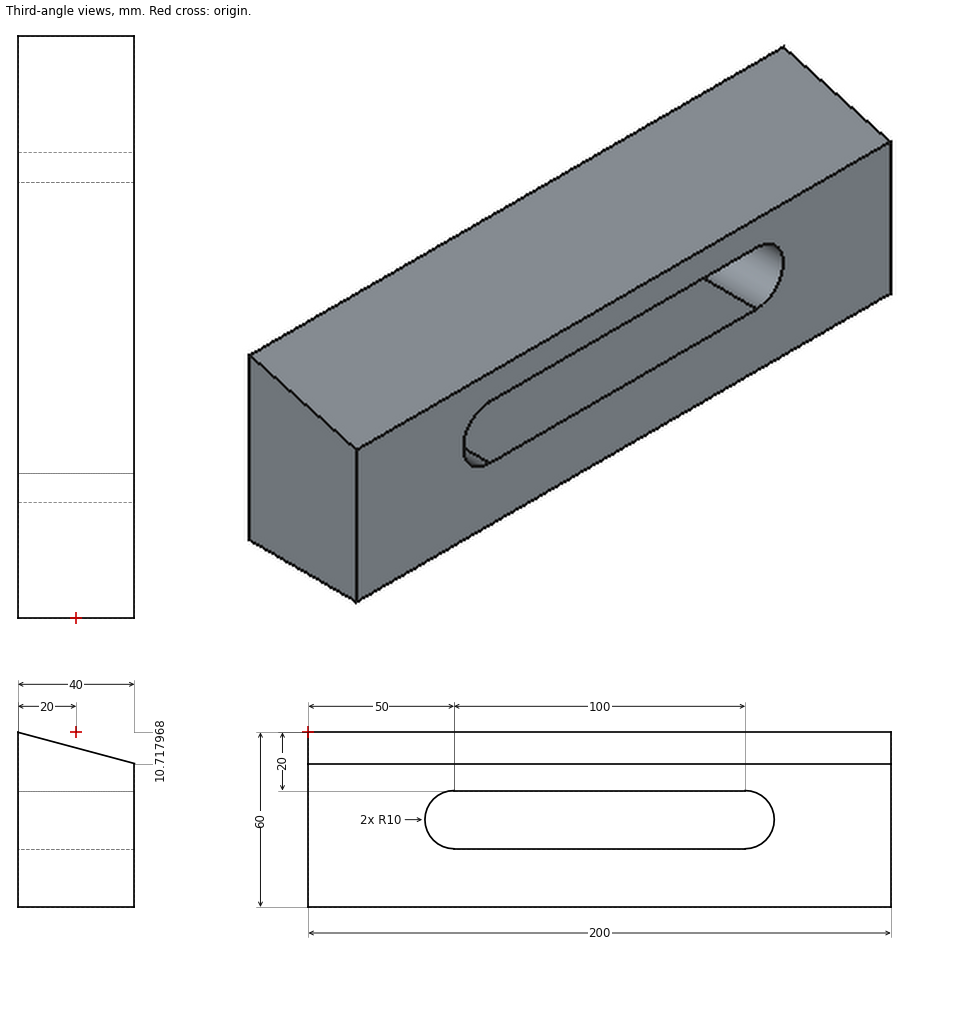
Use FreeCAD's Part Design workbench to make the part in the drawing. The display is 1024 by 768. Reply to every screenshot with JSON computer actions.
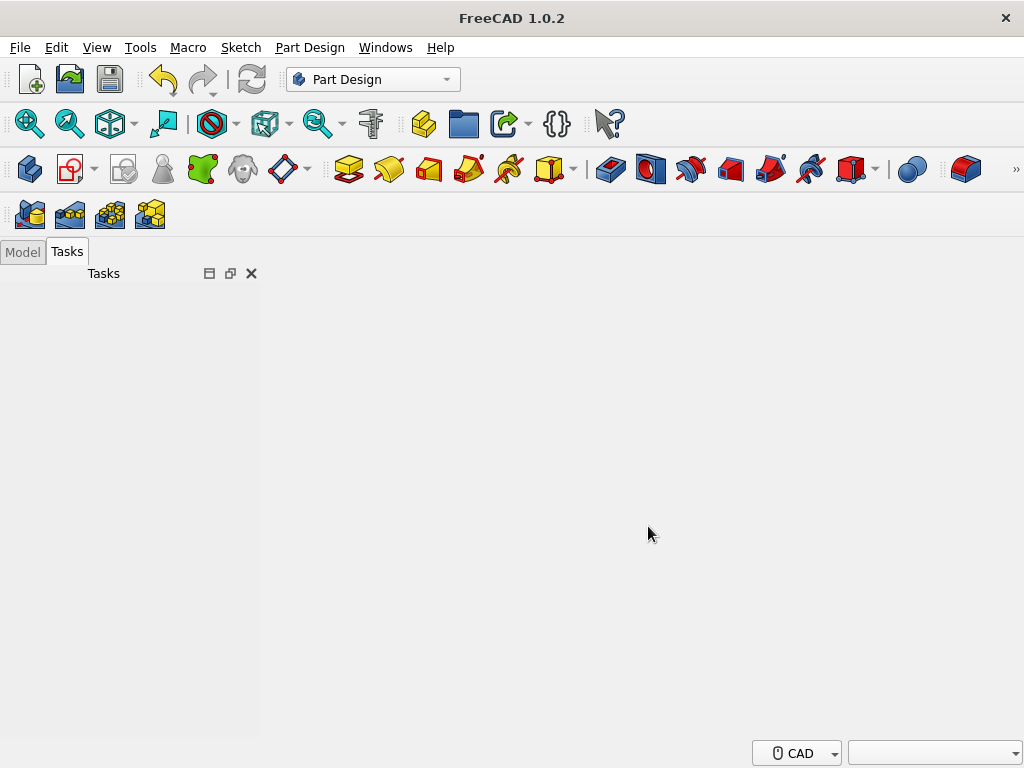
{"action": "left_click", "coordinate": [30, 80]}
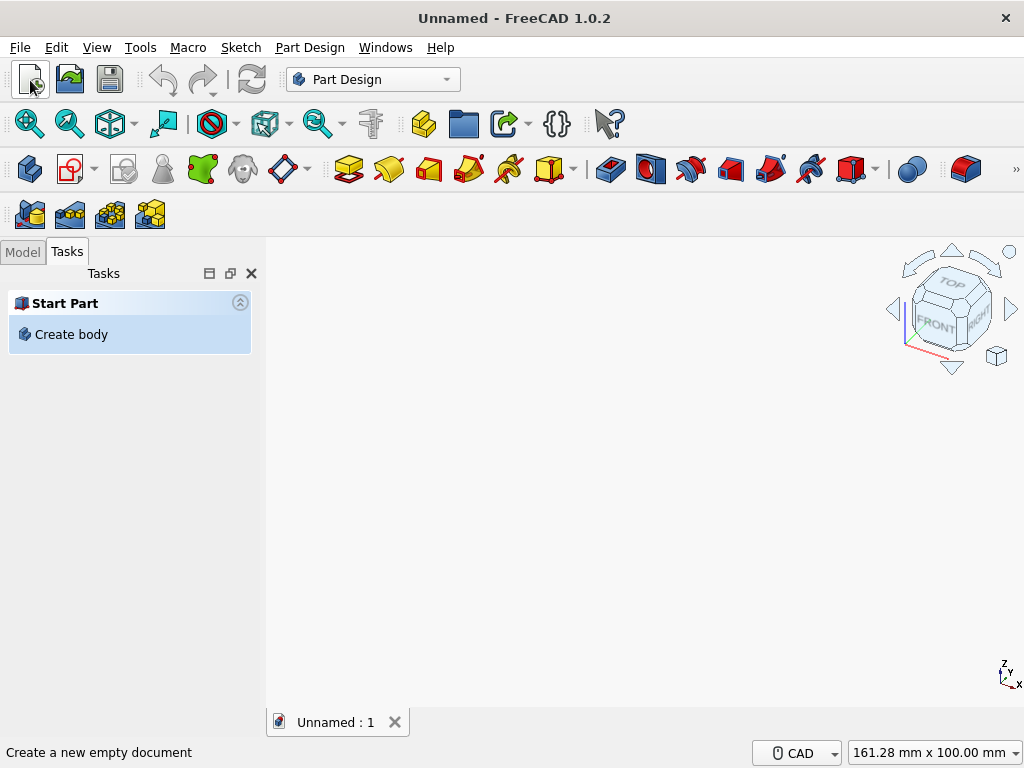
{"action": "left_click", "coordinate": [70, 170]}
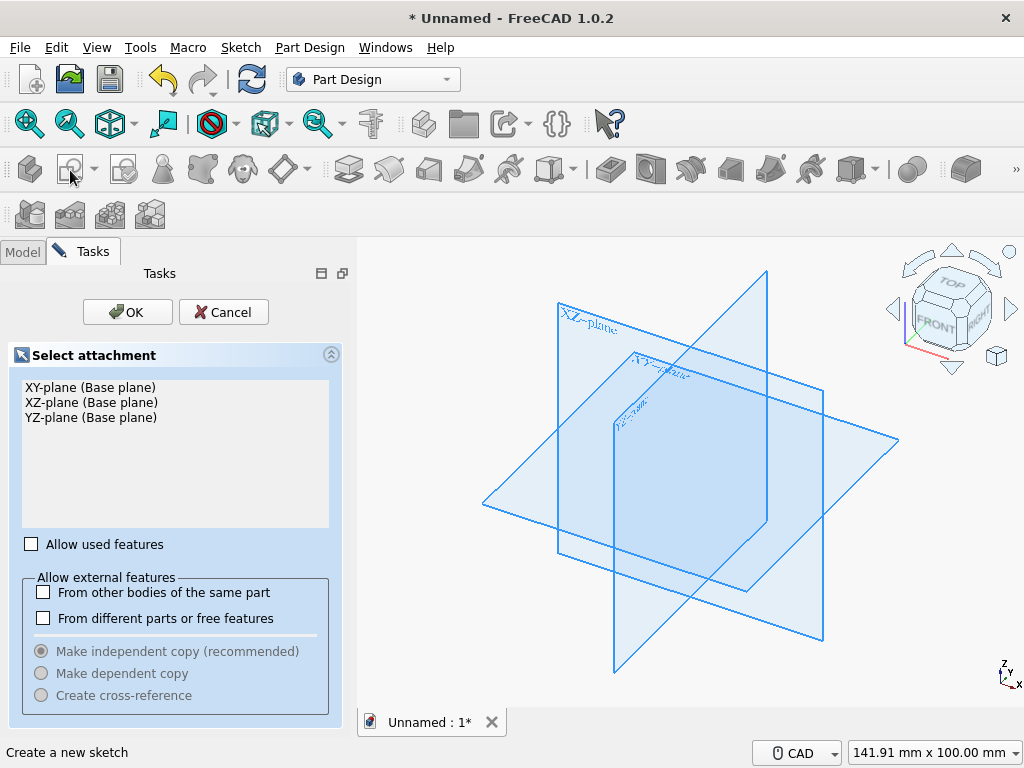
{"action": "left_click", "coordinate": [82, 418]}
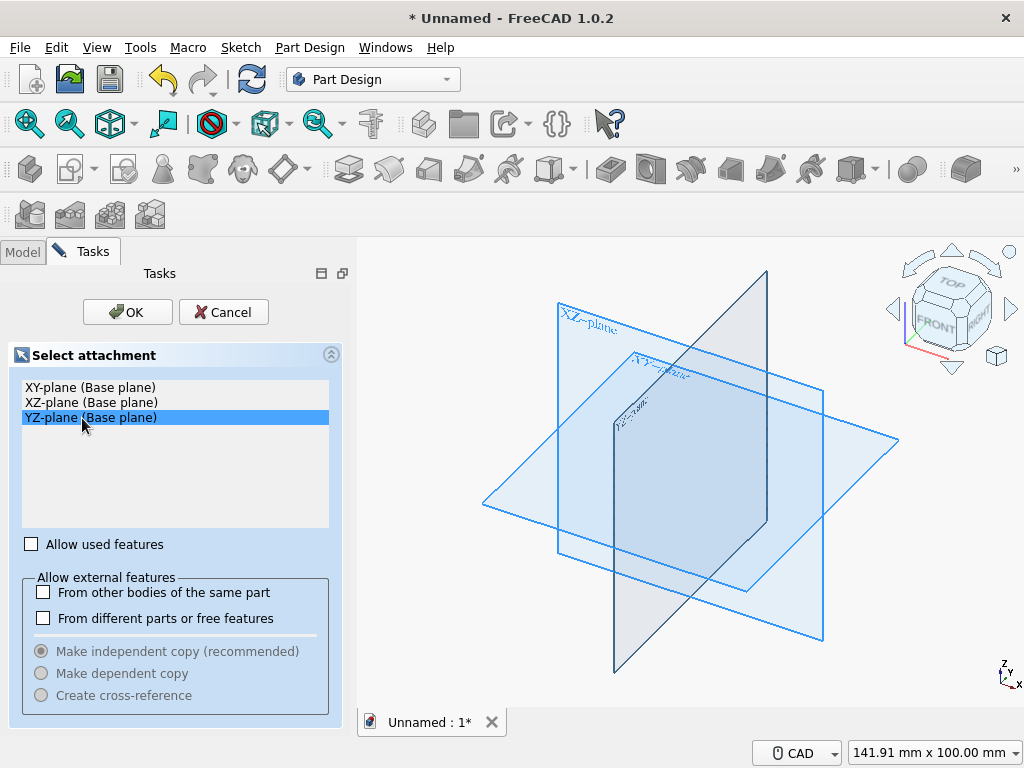
{"action": "left_click", "coordinate": [128, 312]}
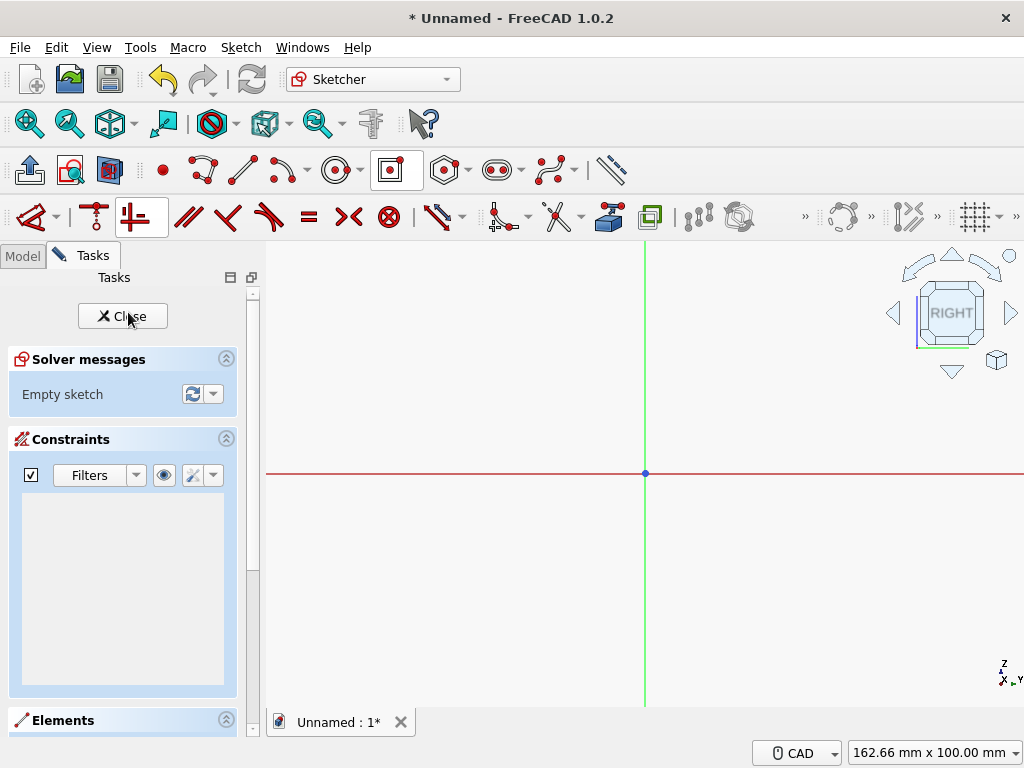
{"action": "scroll", "coordinate": [294, 393], "scroll_direction": "down", "scroll_amount": 5}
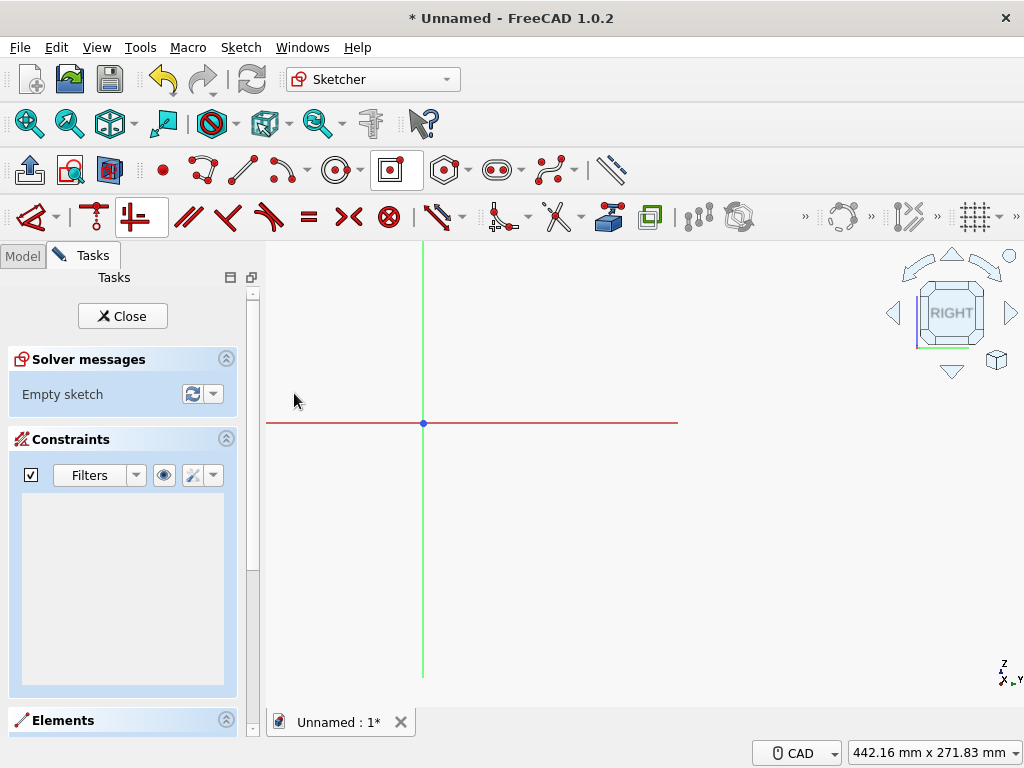
{"action": "left_click", "coordinate": [418, 170]}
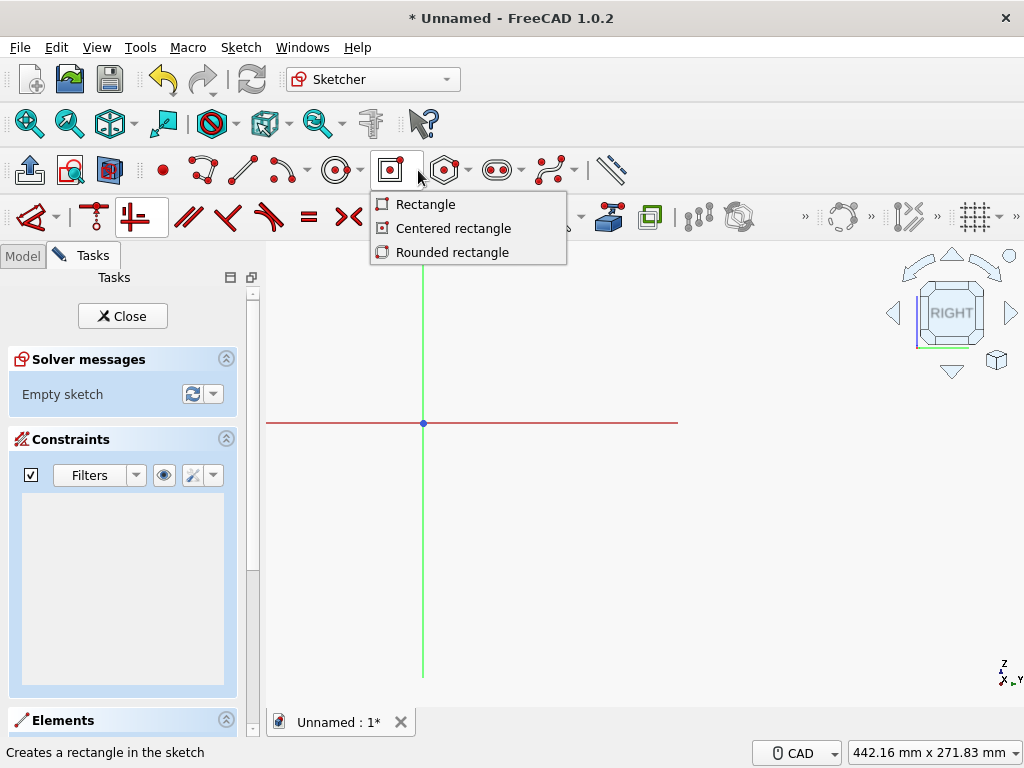
{"action": "left_click", "coordinate": [468, 204]}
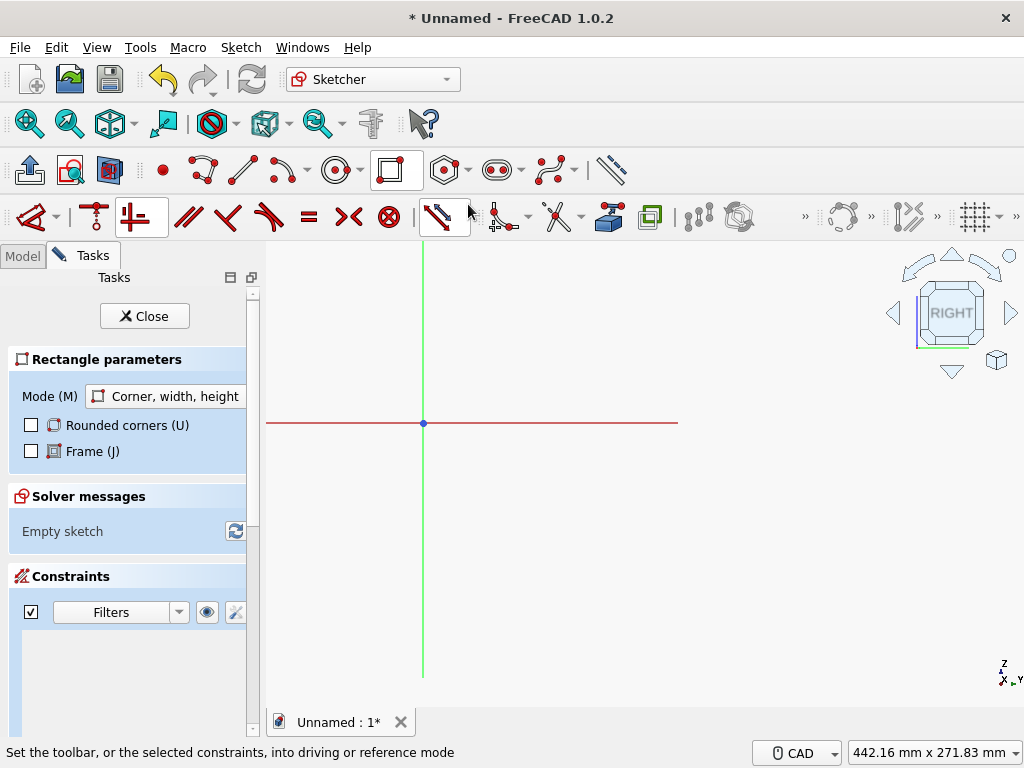
{"action": "left_click", "coordinate": [423, 423]}
{"action": "left_click", "coordinate": [766, 526]}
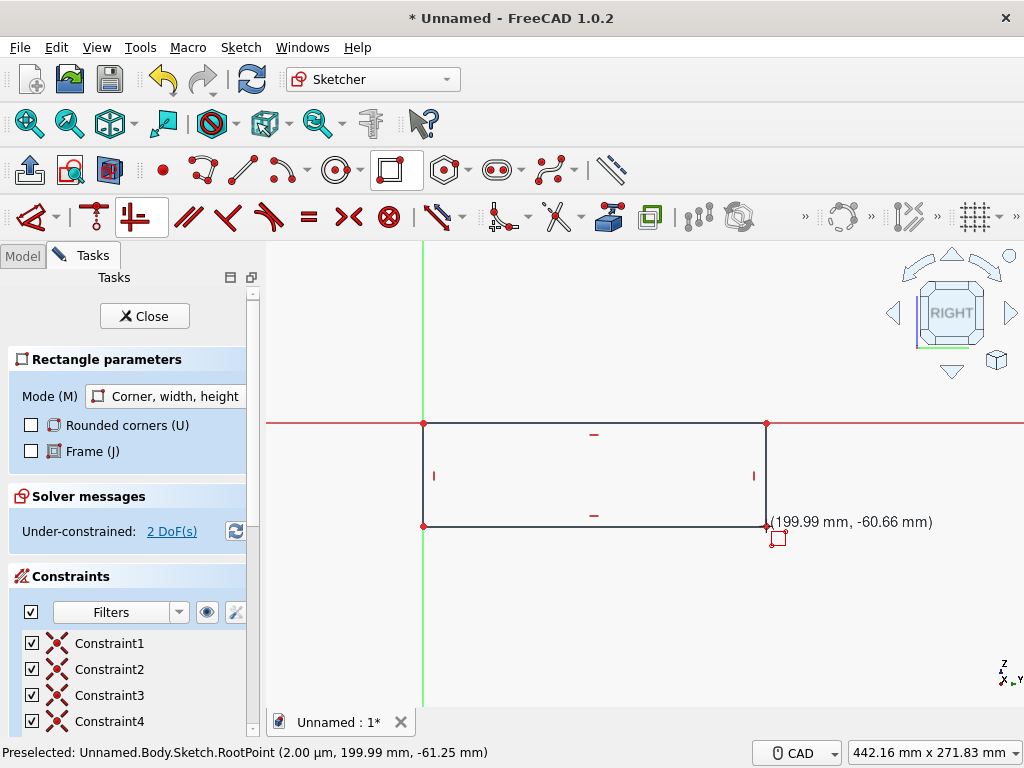
{"action": "left_click", "coordinate": [498, 170]}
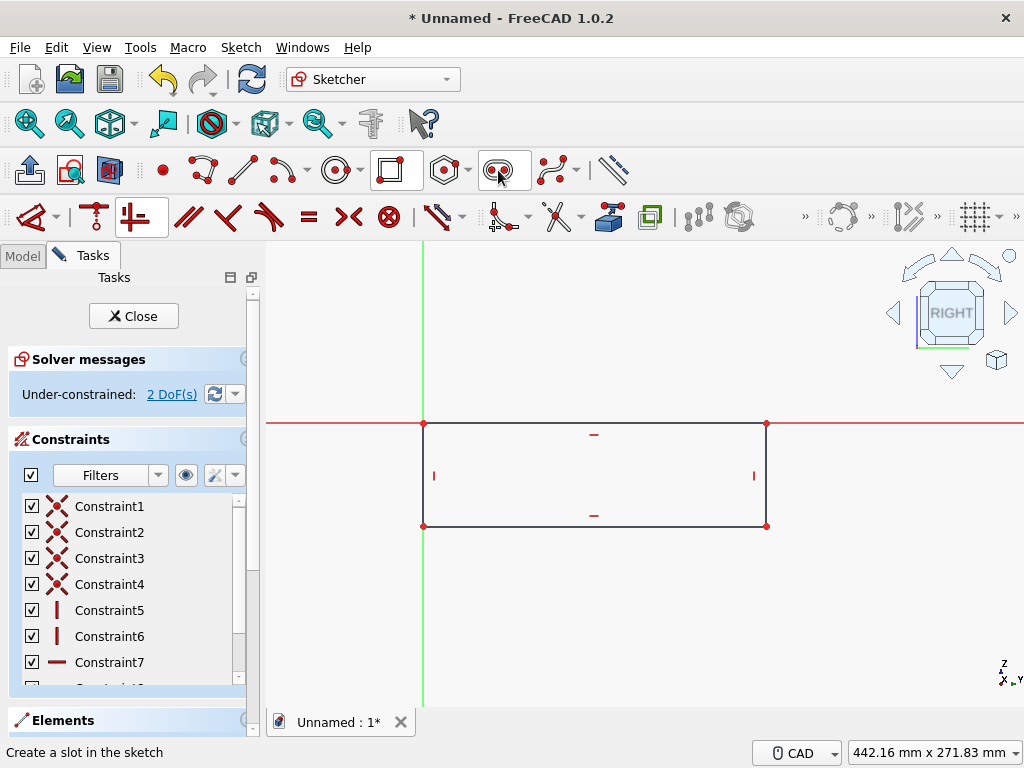
{"action": "scroll", "coordinate": [509, 474], "scroll_direction": "up", "scroll_amount": 2}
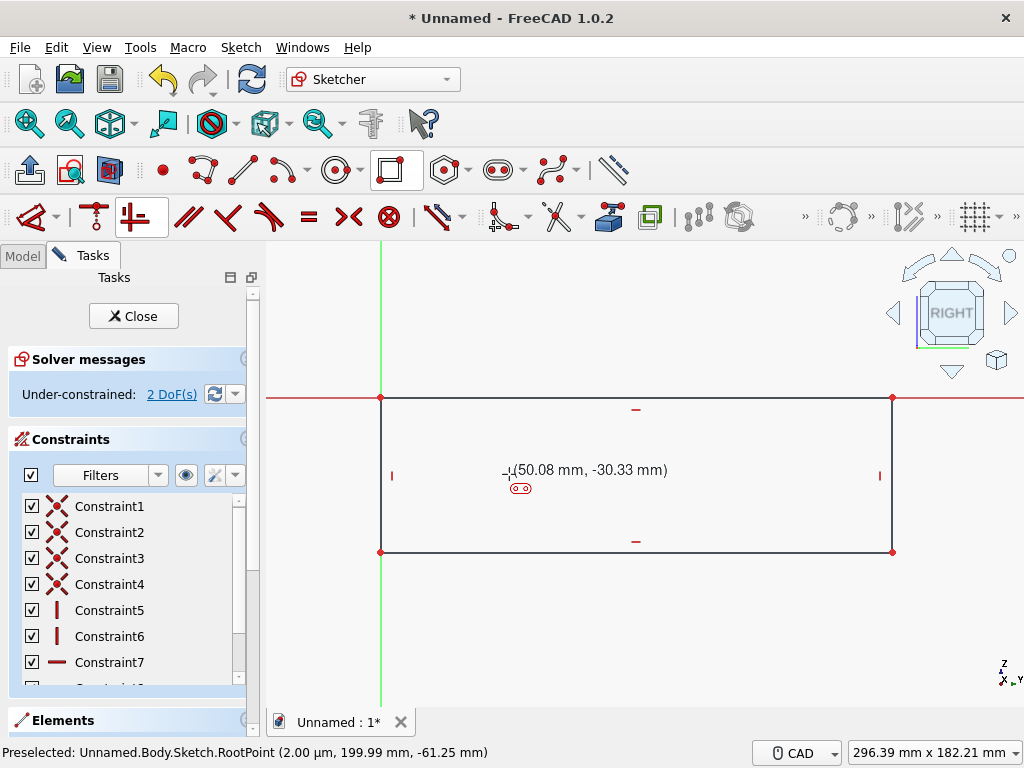
{"action": "left_click", "coordinate": [509, 474]}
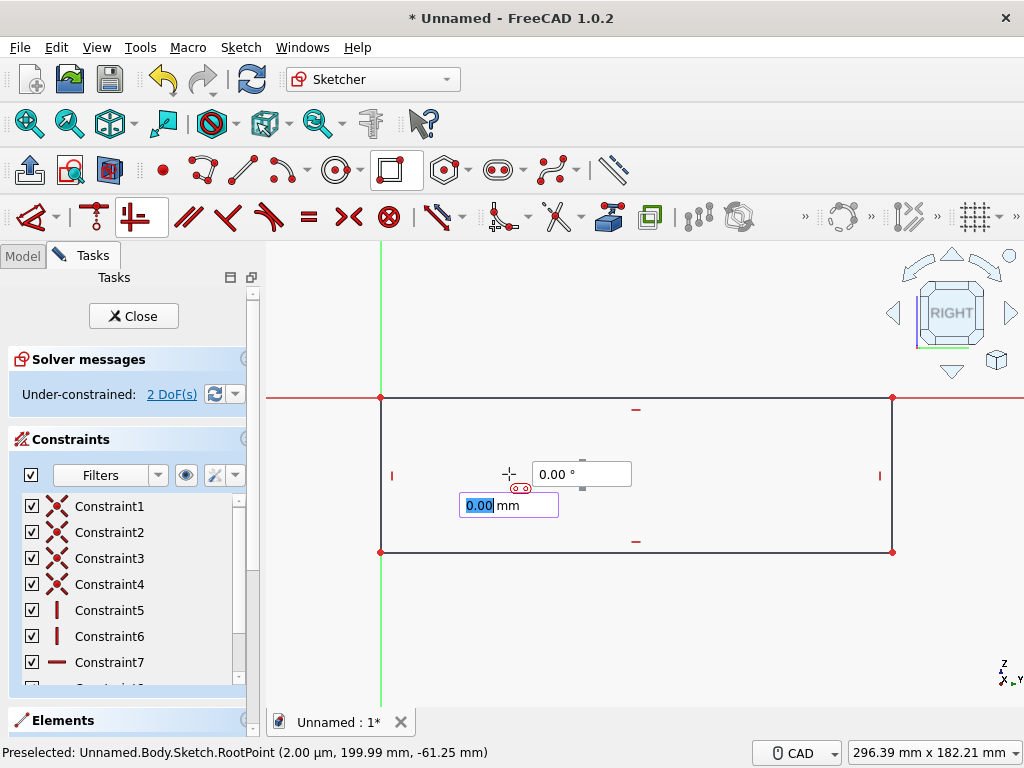
{"action": "left_click", "coordinate": [764, 474]}